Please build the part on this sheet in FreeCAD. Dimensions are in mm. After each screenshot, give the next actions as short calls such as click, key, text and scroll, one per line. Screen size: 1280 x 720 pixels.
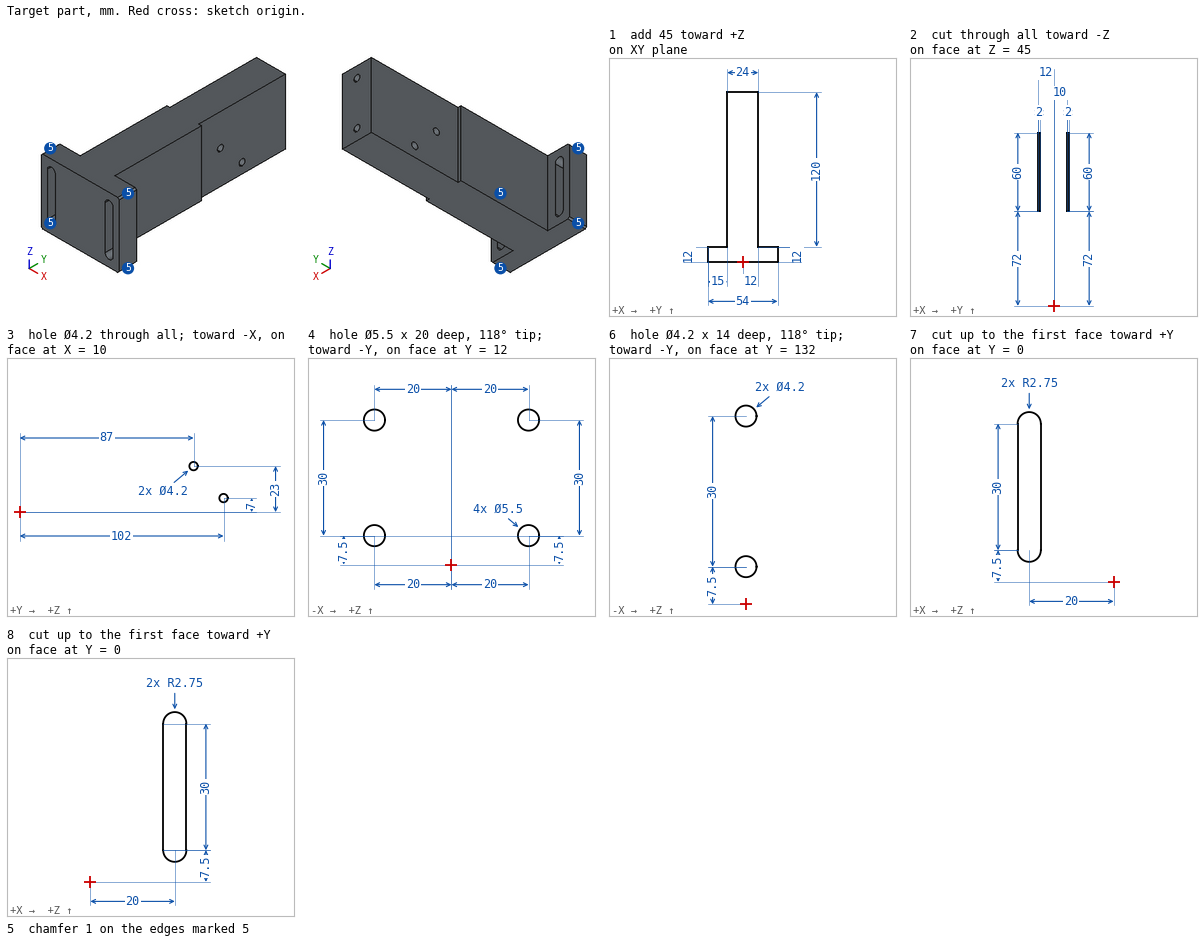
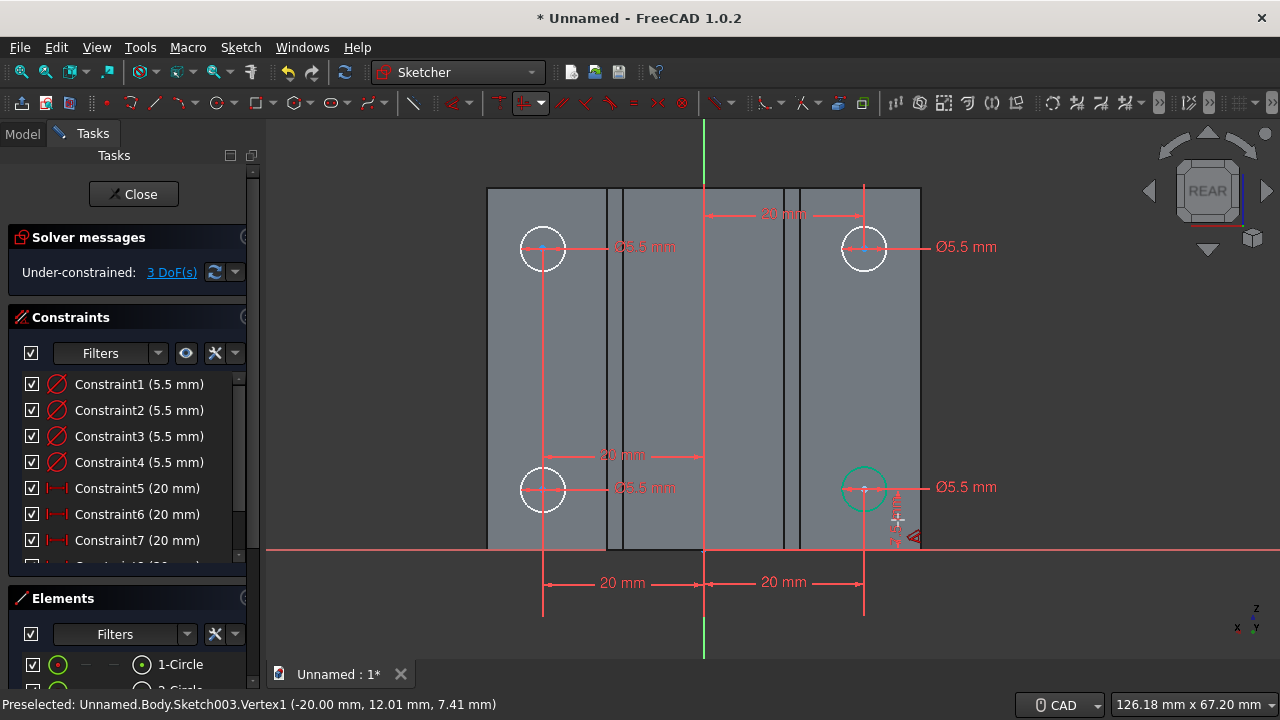
click(543, 490)
click(509, 520)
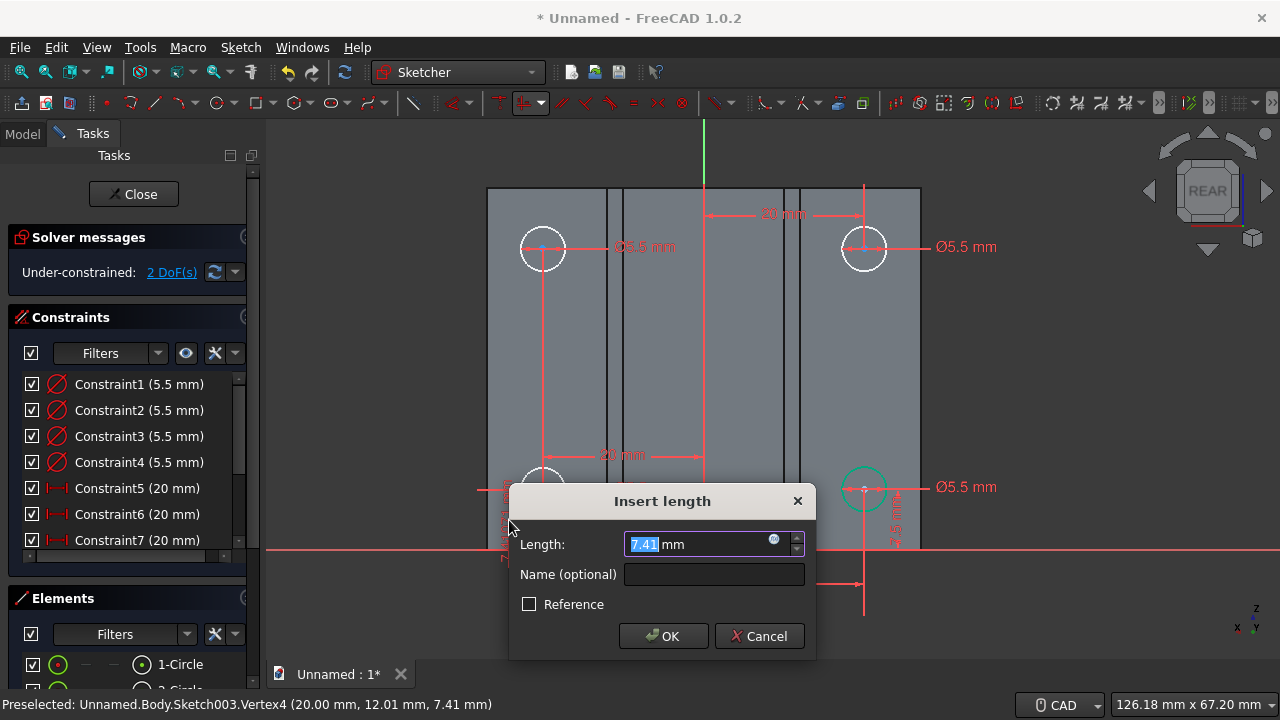
text(7.5)
key(Return)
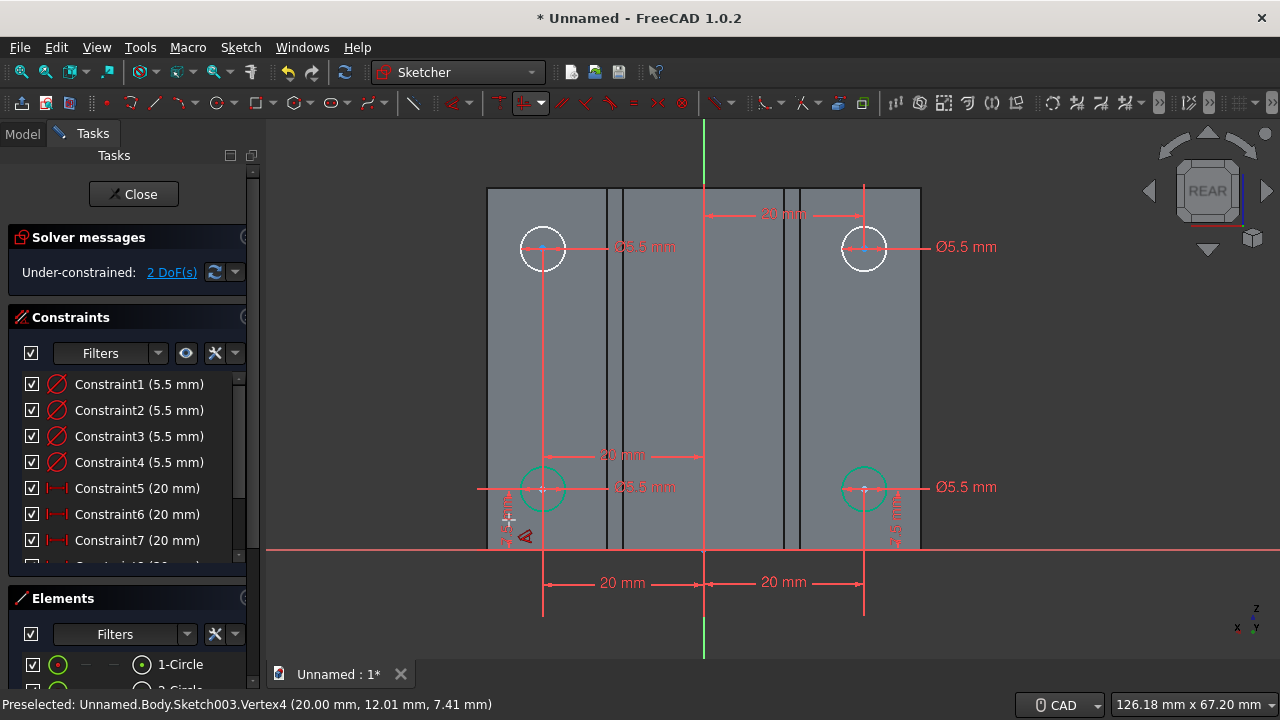
click(864, 489)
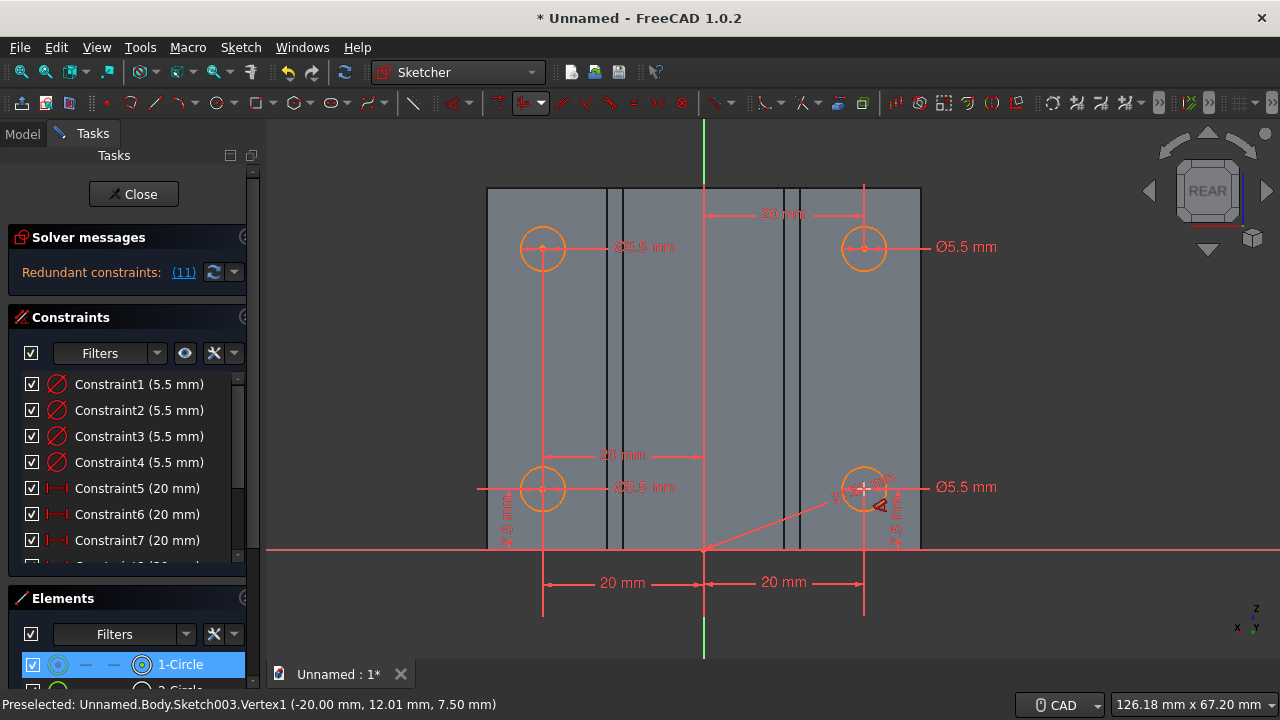
click(864, 249)
click(898, 369)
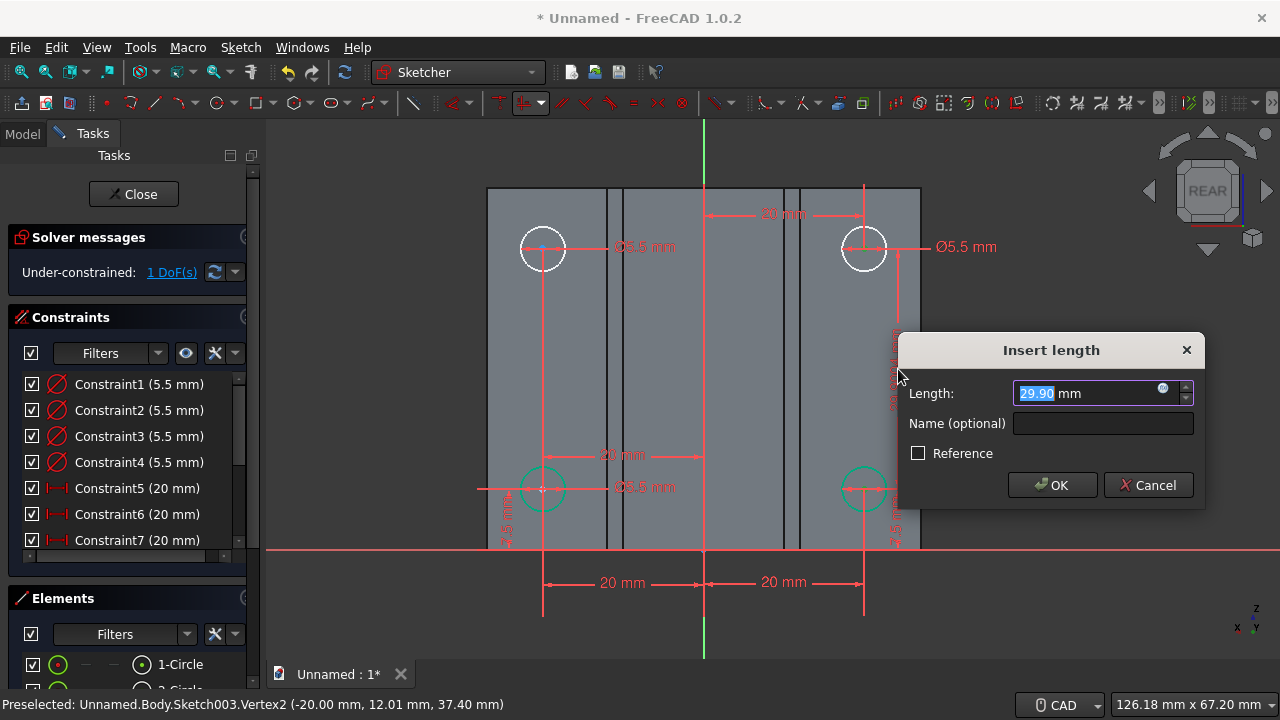
text(30)
key(Return)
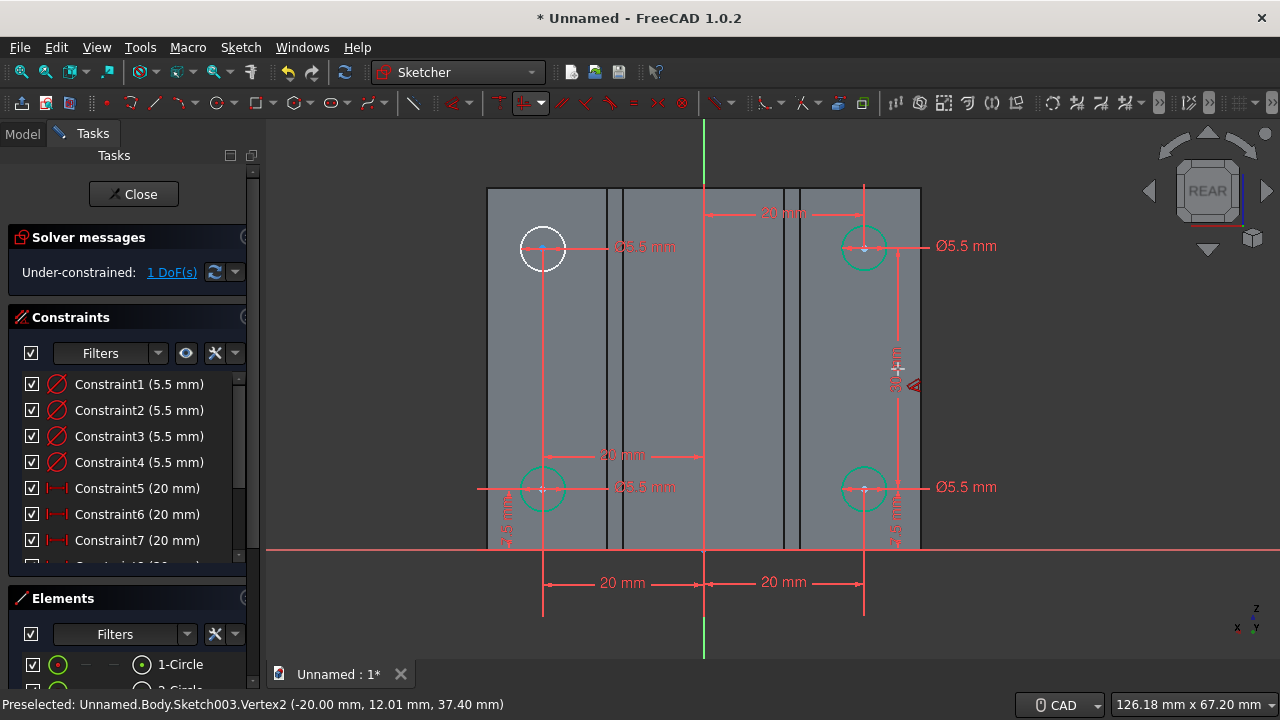
click(864, 489)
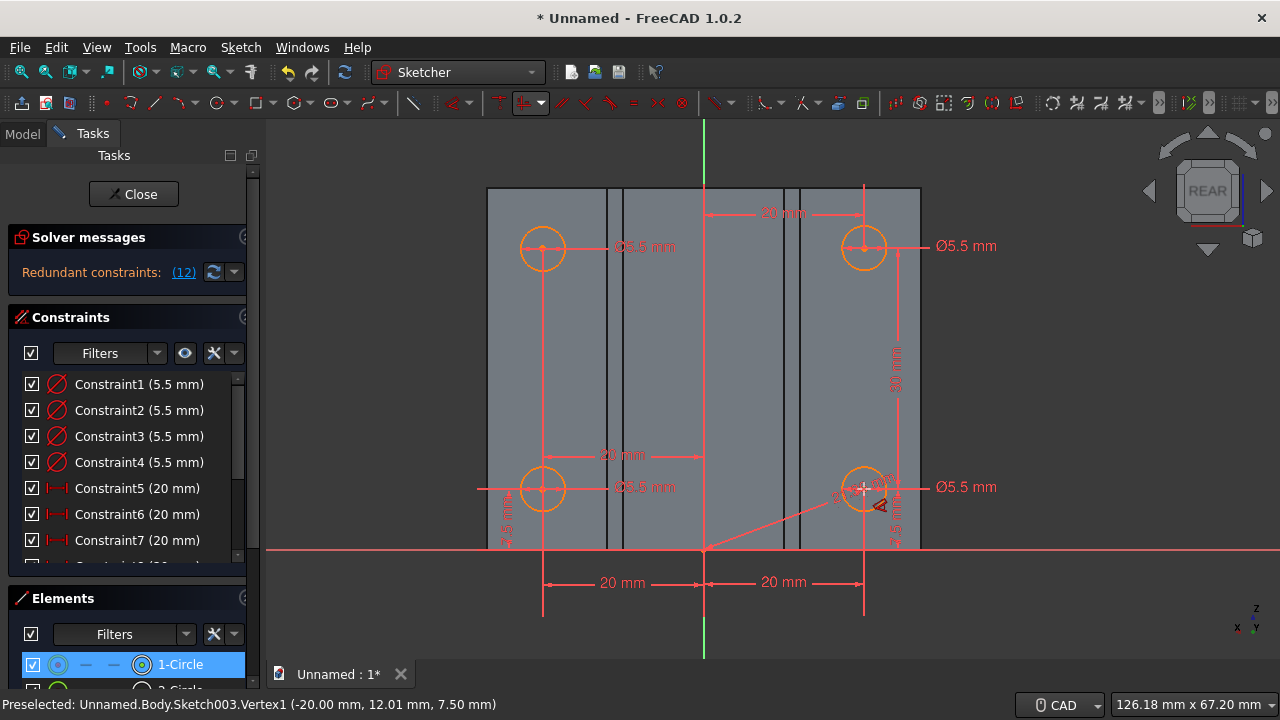
click(543, 249)
click(898, 314)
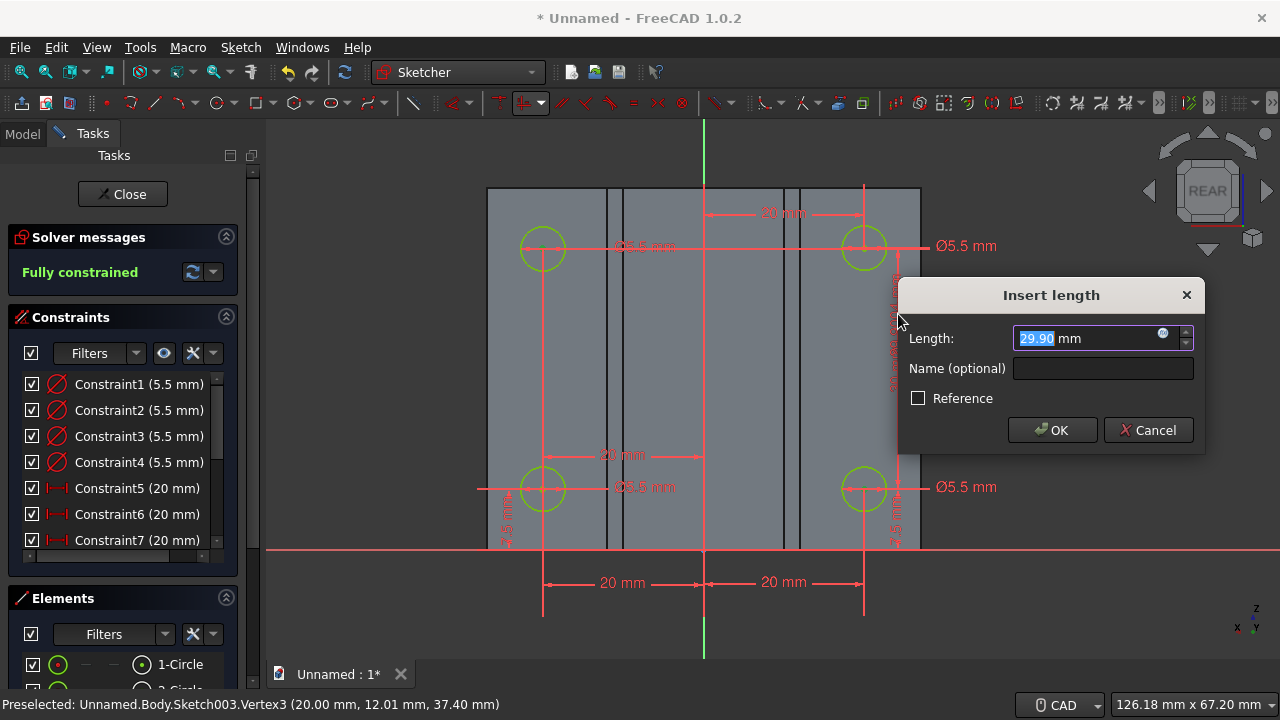
text(30)
key(Return)
key(Escape)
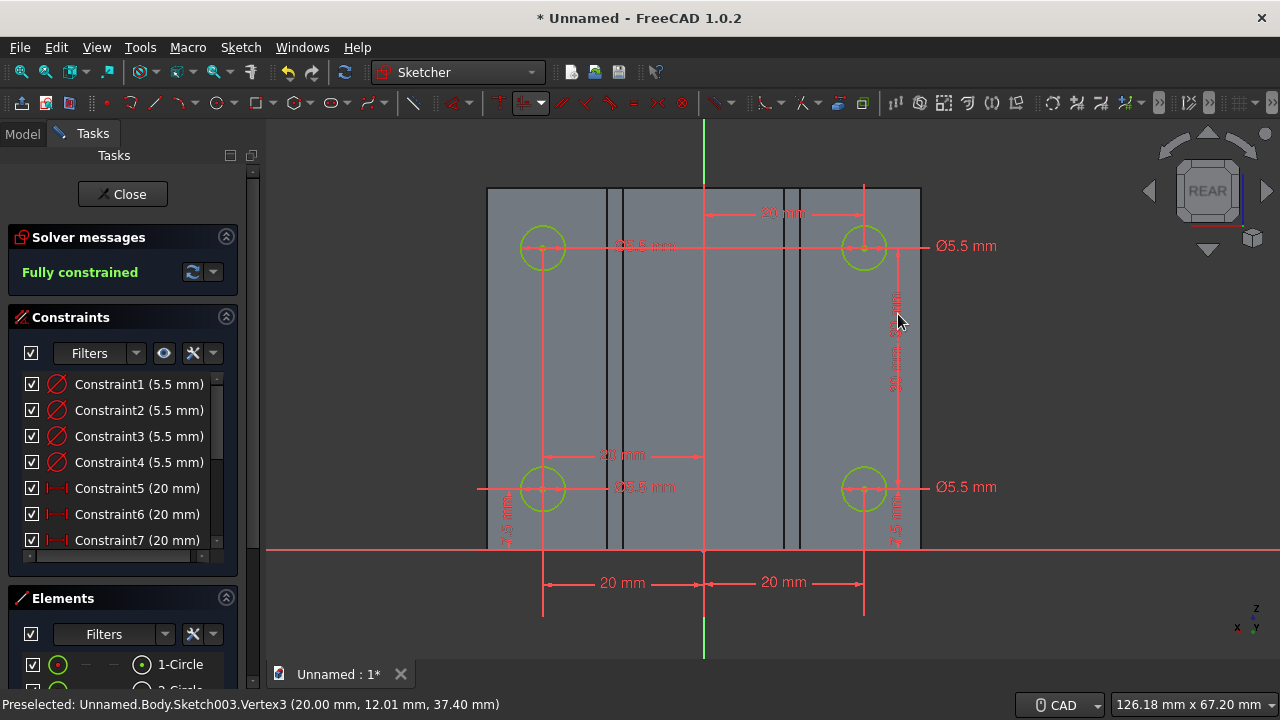
click(123, 194)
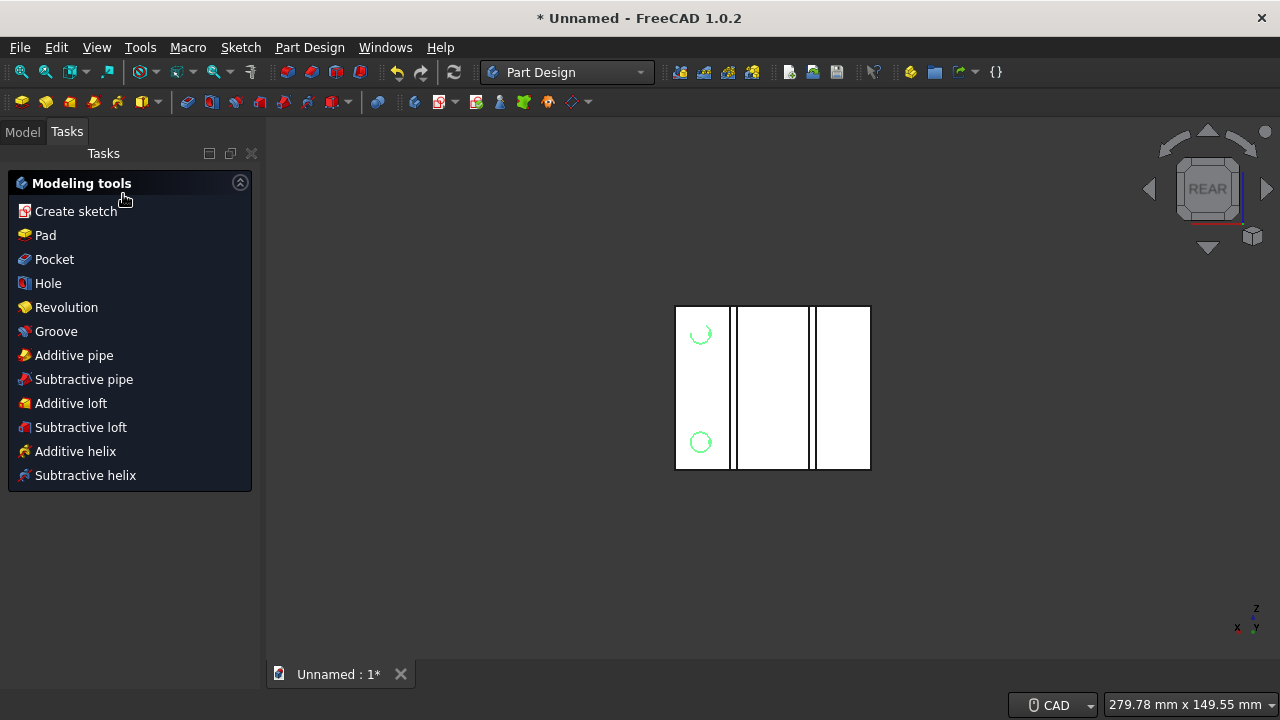
click(212, 102)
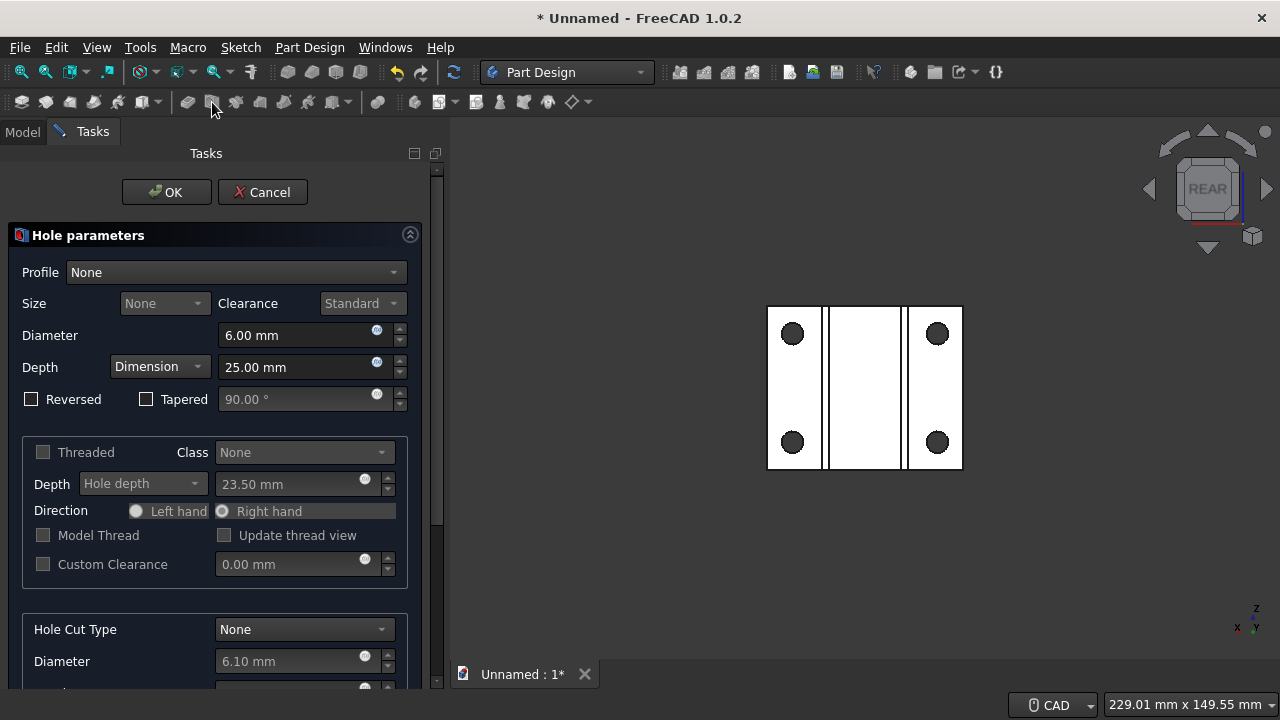
triple_click(305, 335)